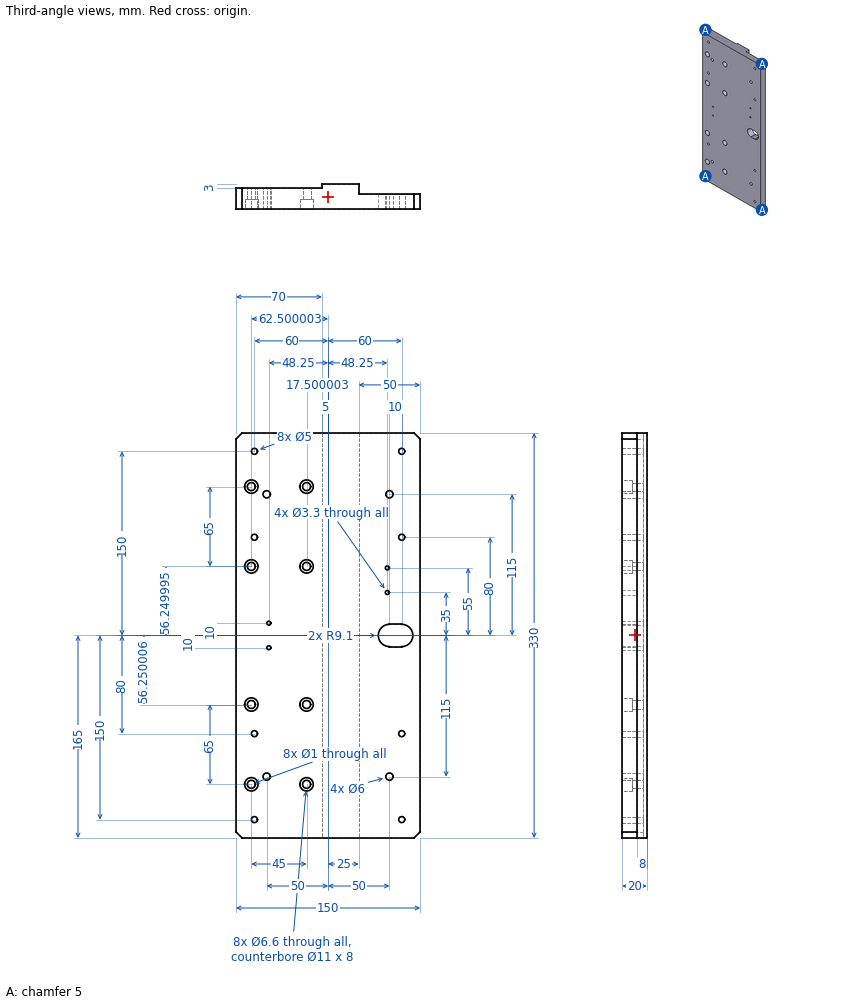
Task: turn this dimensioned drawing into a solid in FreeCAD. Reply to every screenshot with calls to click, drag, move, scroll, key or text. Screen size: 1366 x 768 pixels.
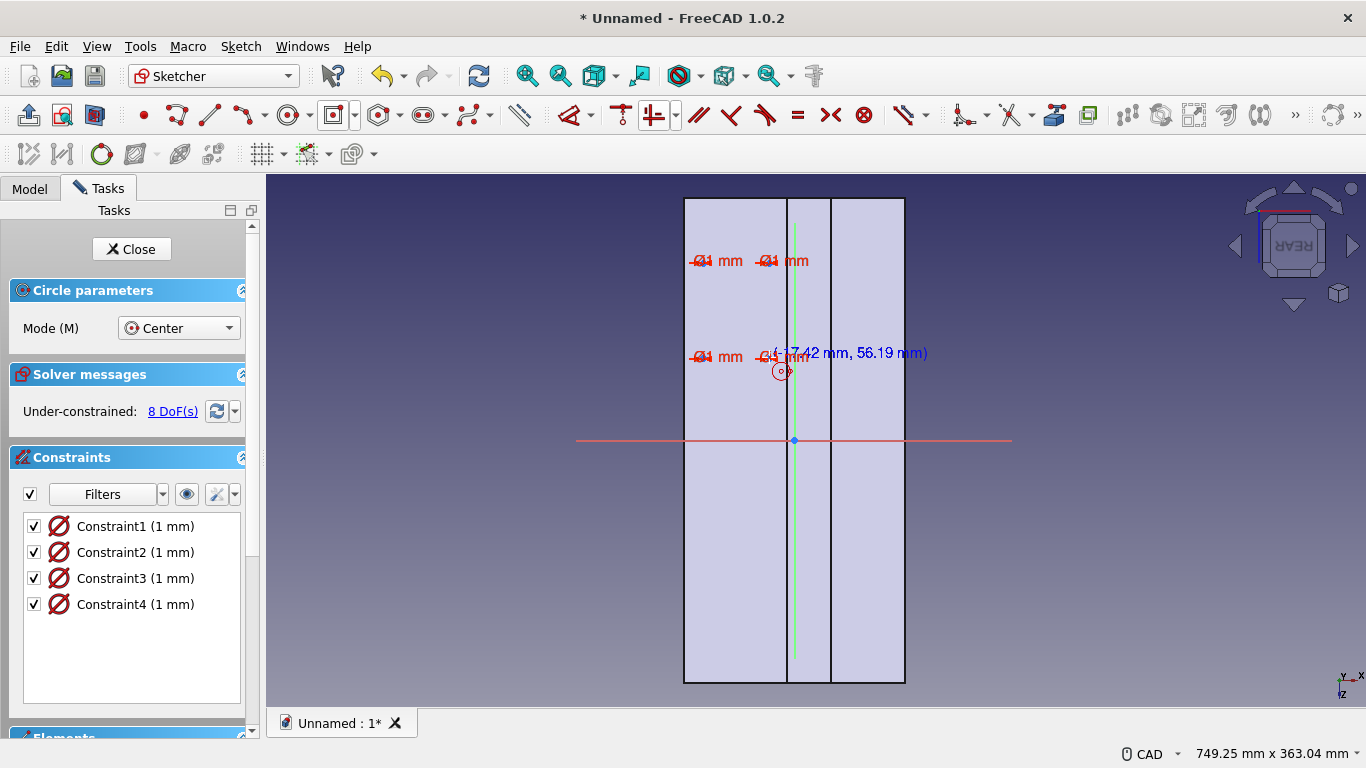
scroll(703, 523, up, 18)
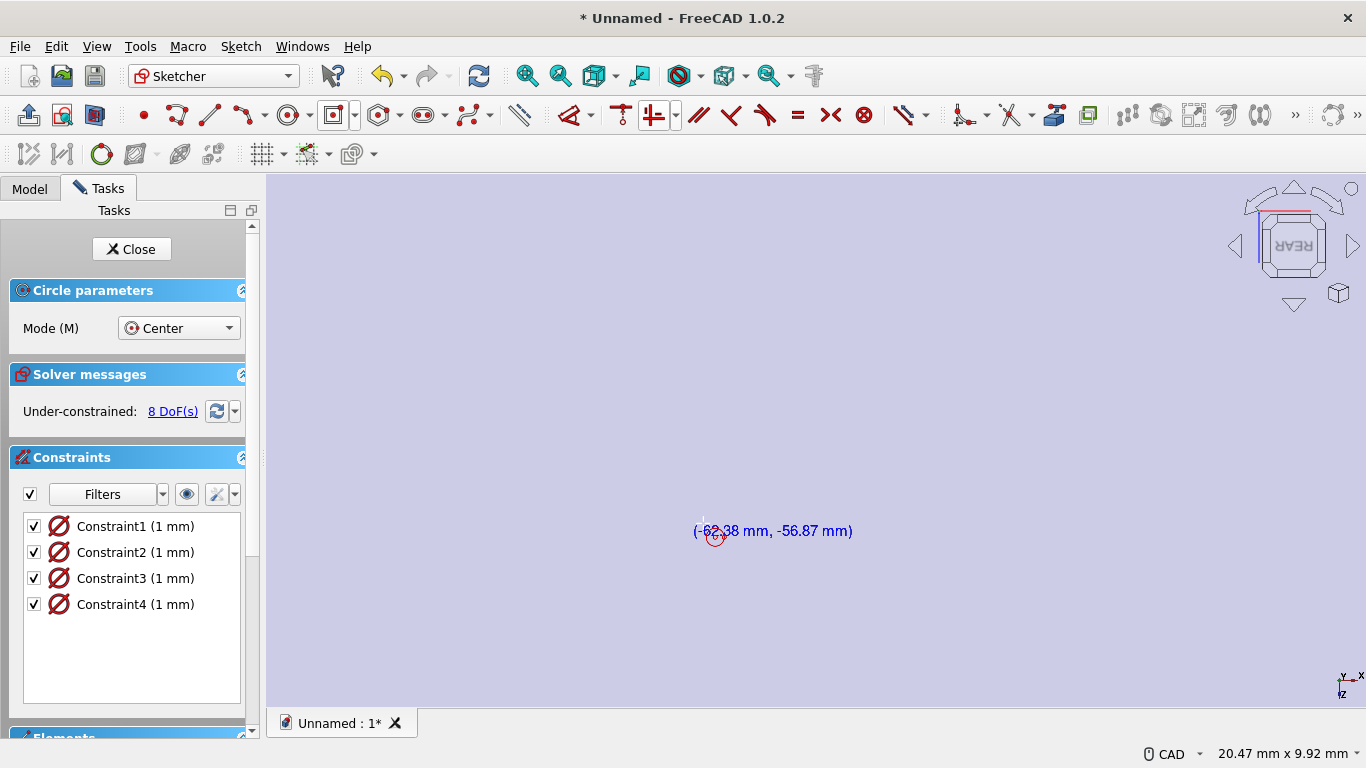
scroll(703, 524, down, 18)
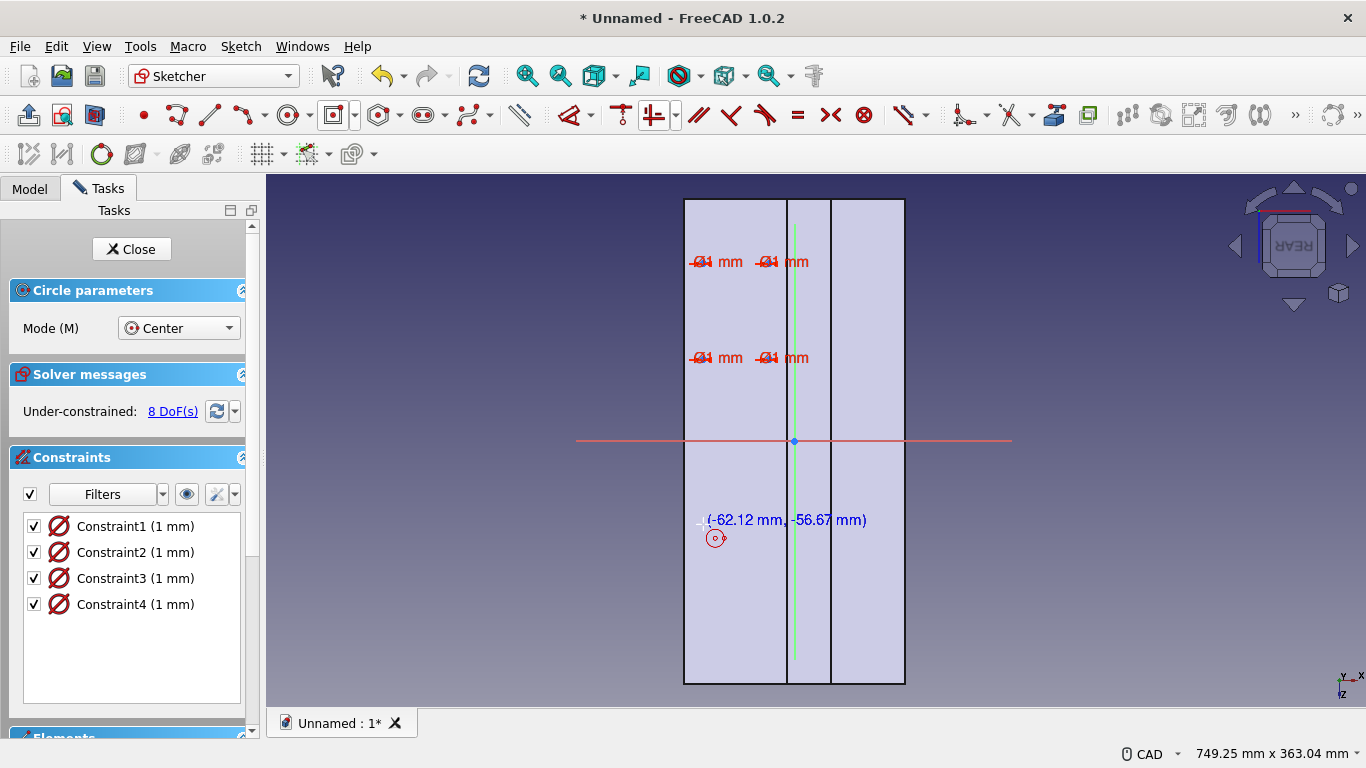
click(703, 524)
move(703, 524)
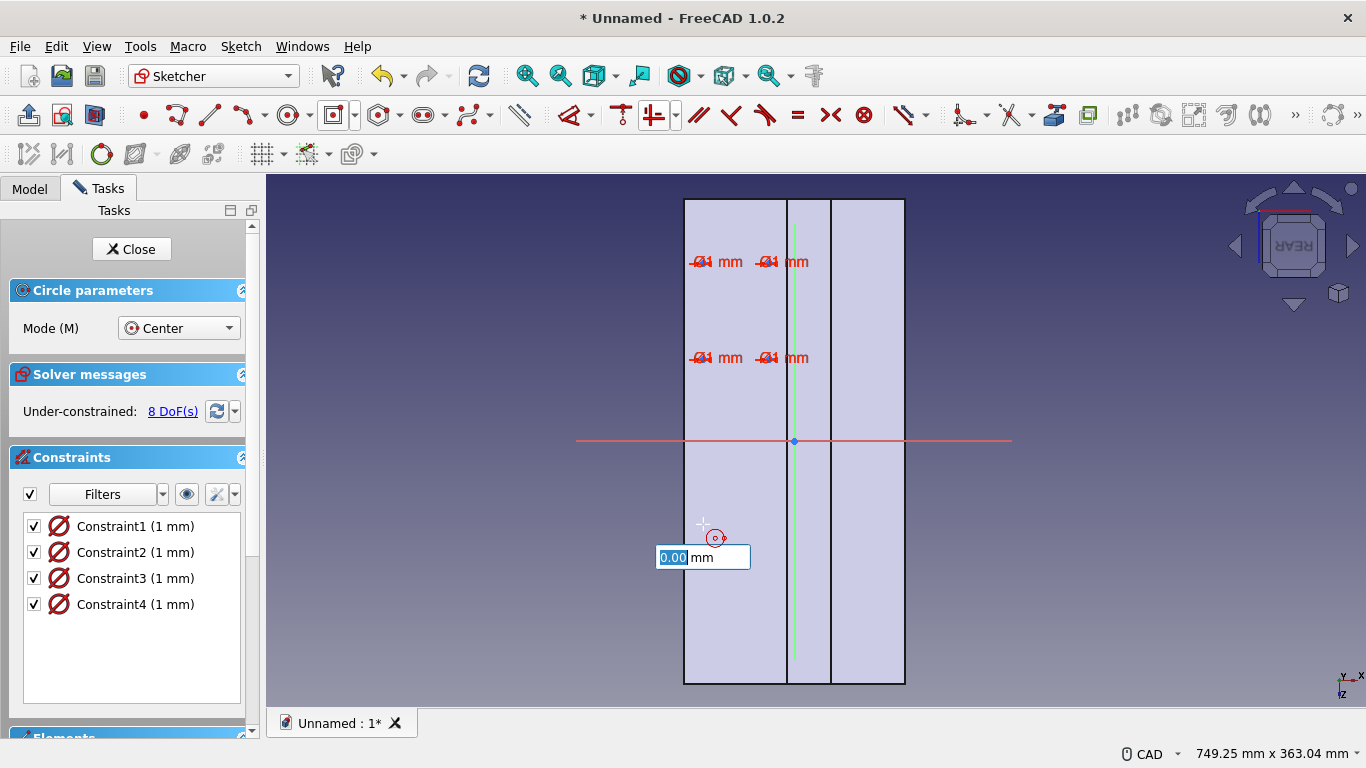
text(1)
key(Return)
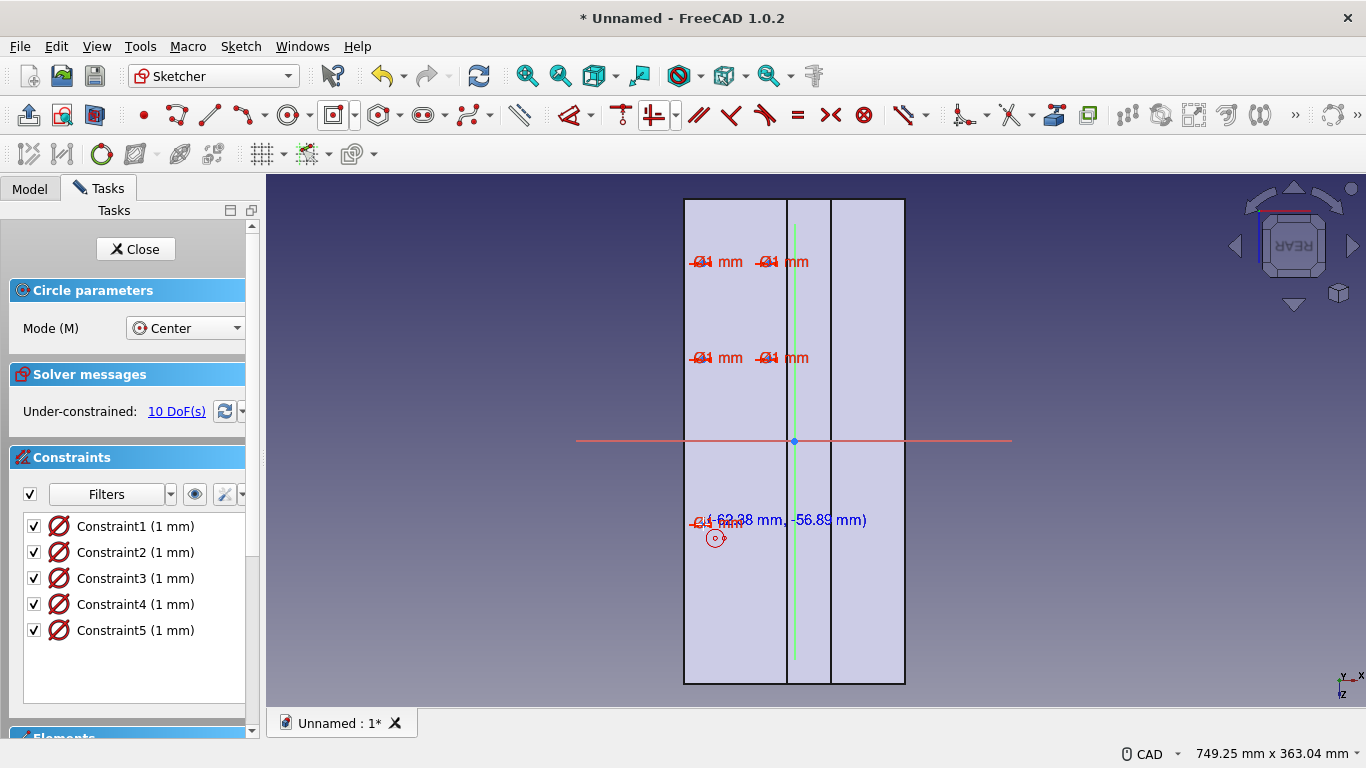
scroll(769, 524, up, 18)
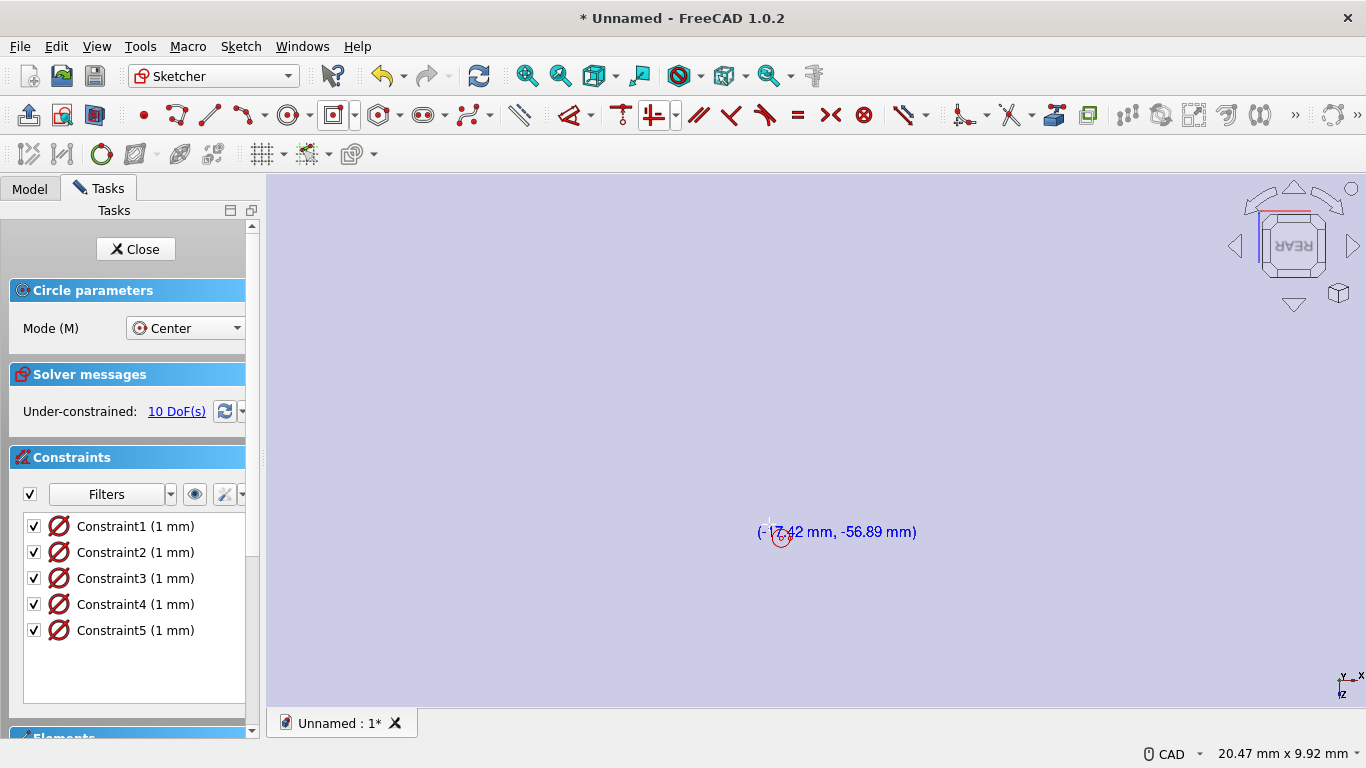
scroll(769, 524, down, 18)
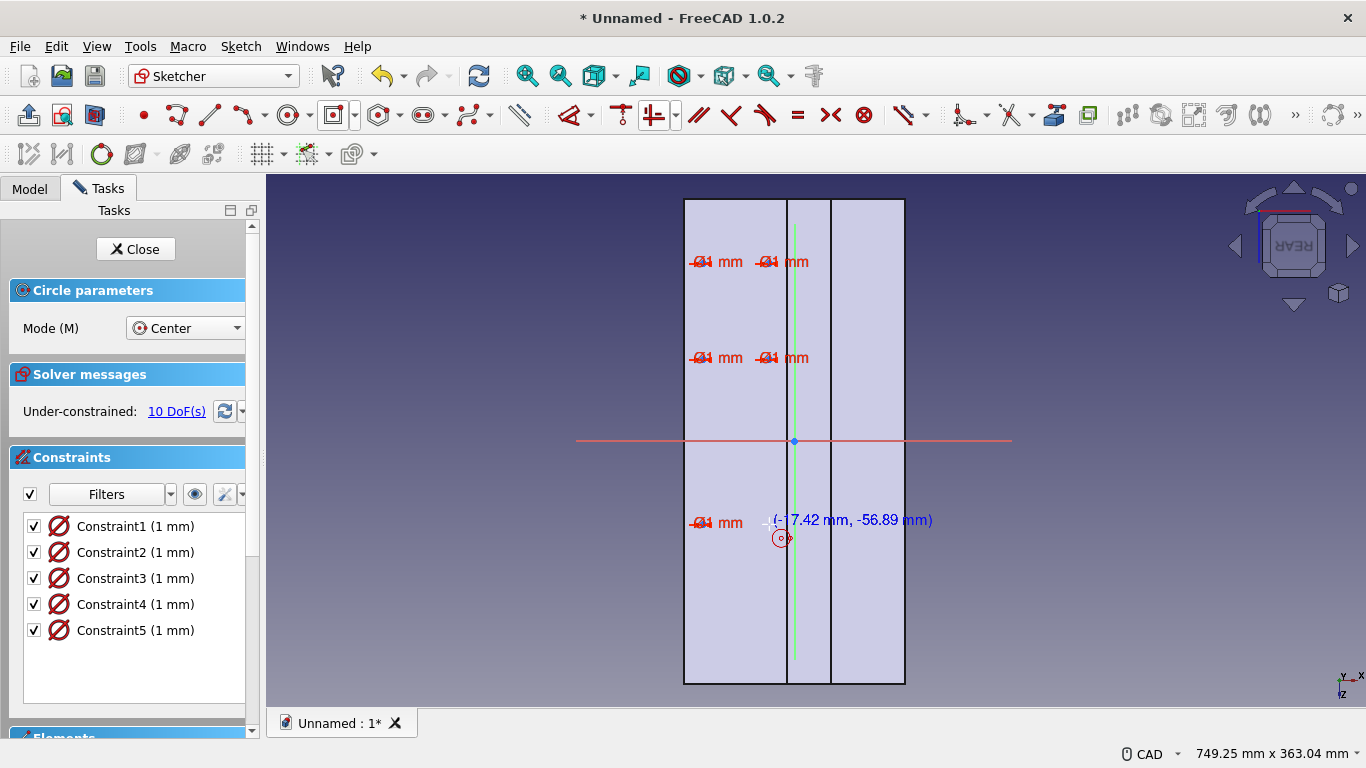
click(769, 524)
move(769, 524)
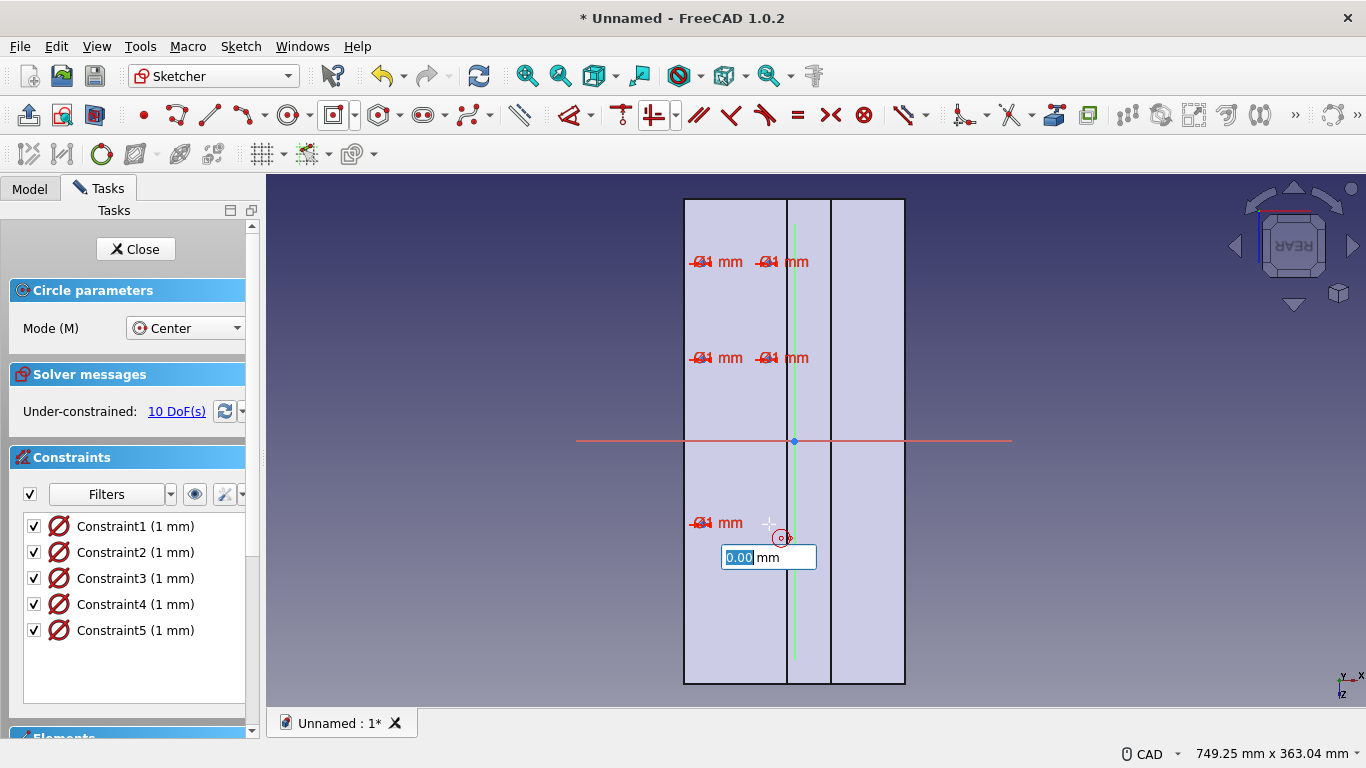
text(1)
key(Return)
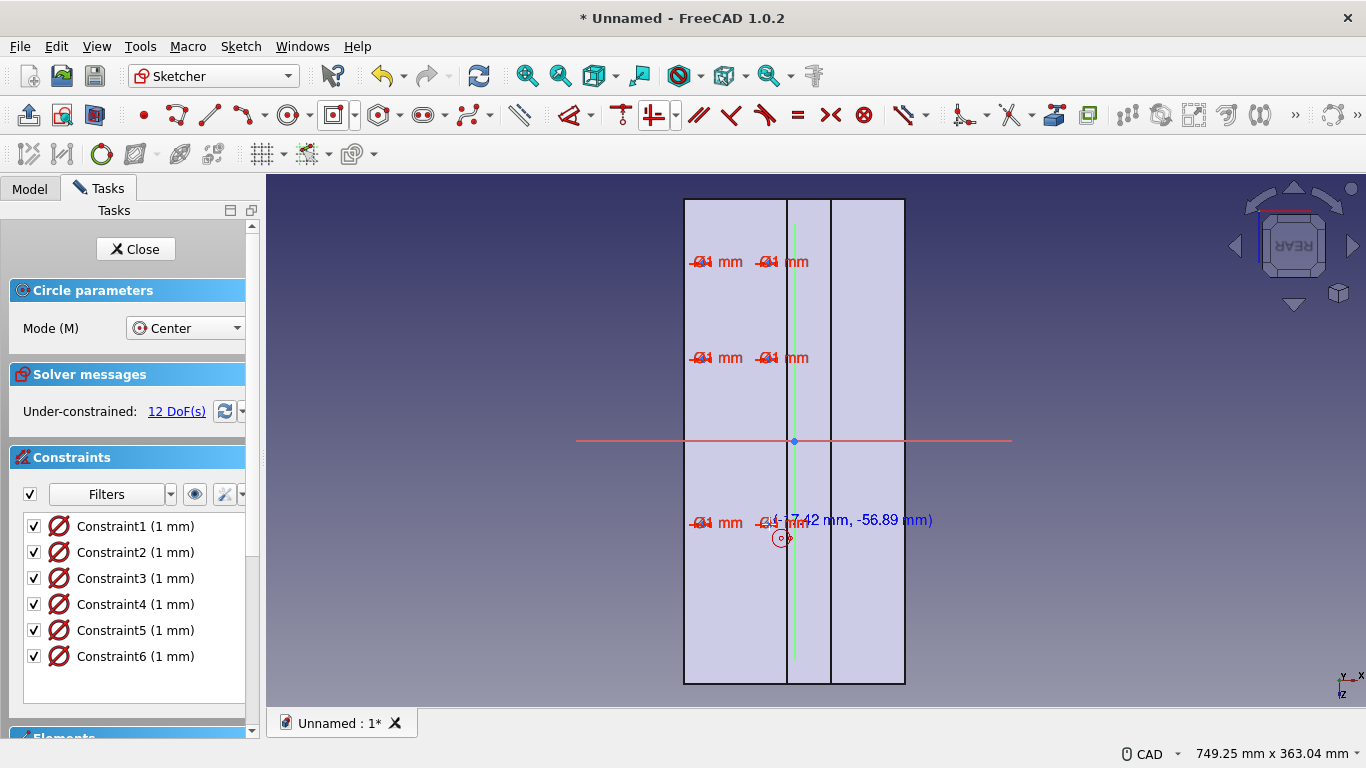
scroll(703, 619, up, 18)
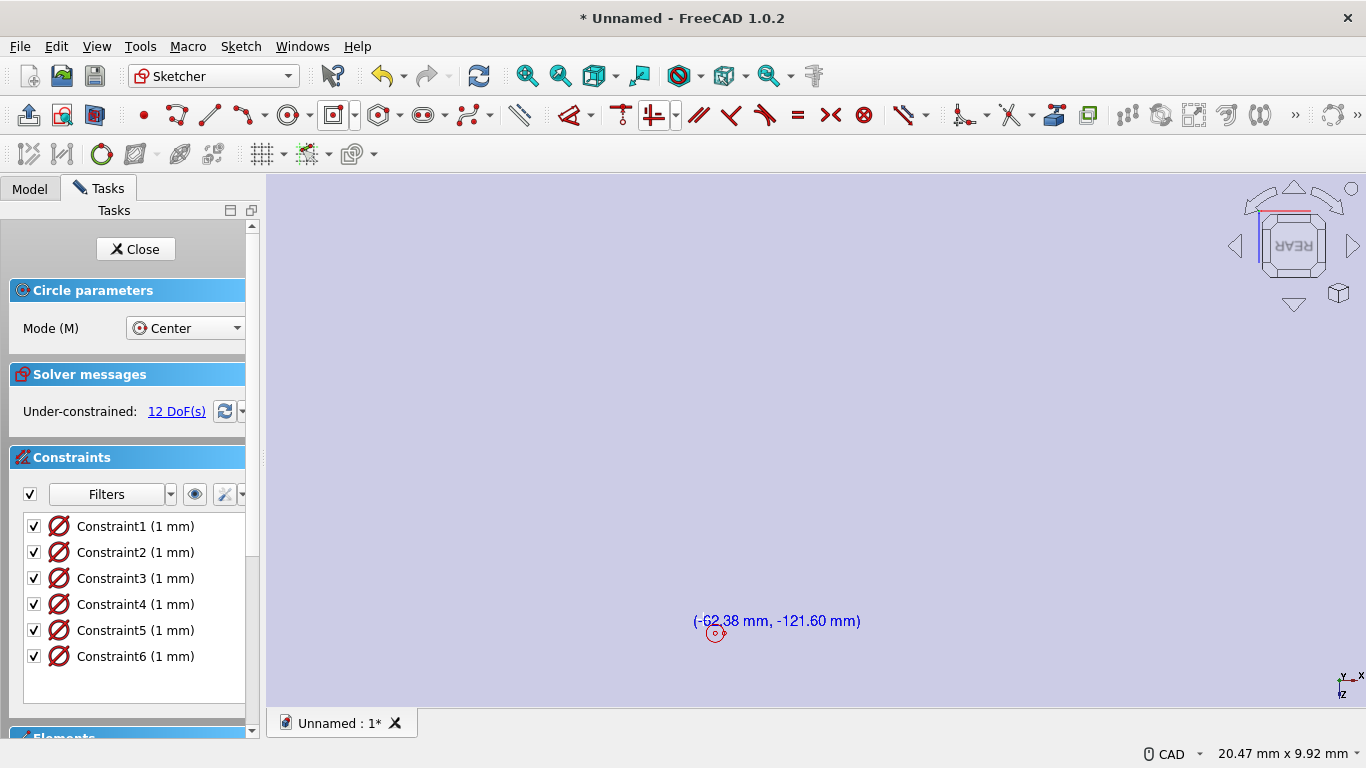
scroll(703, 619, down, 18)